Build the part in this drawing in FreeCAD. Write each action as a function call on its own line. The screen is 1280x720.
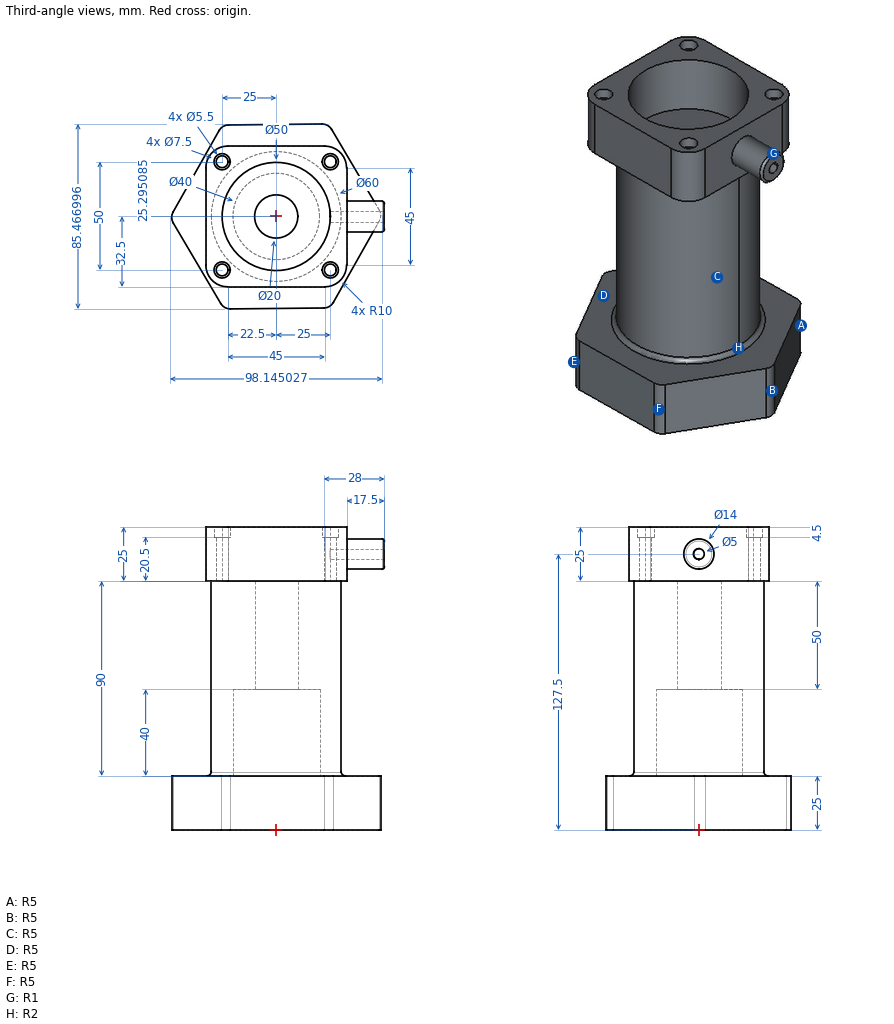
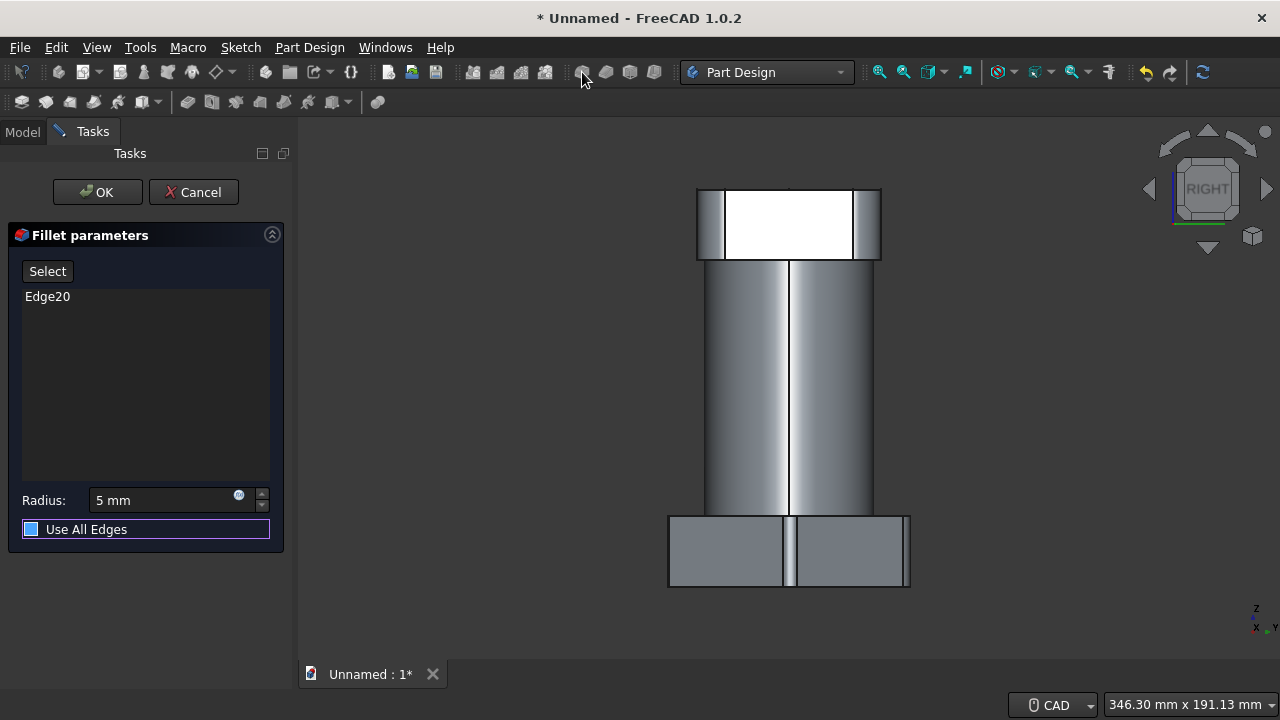
click(98, 192)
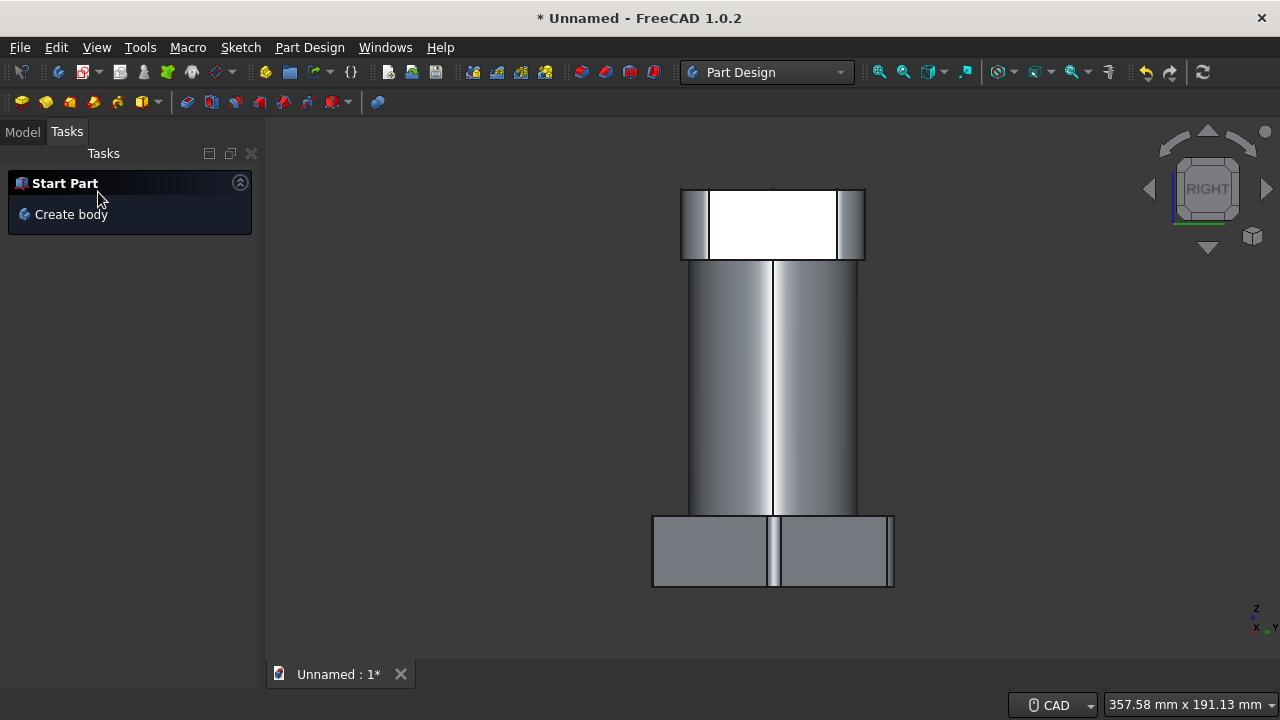
key(0)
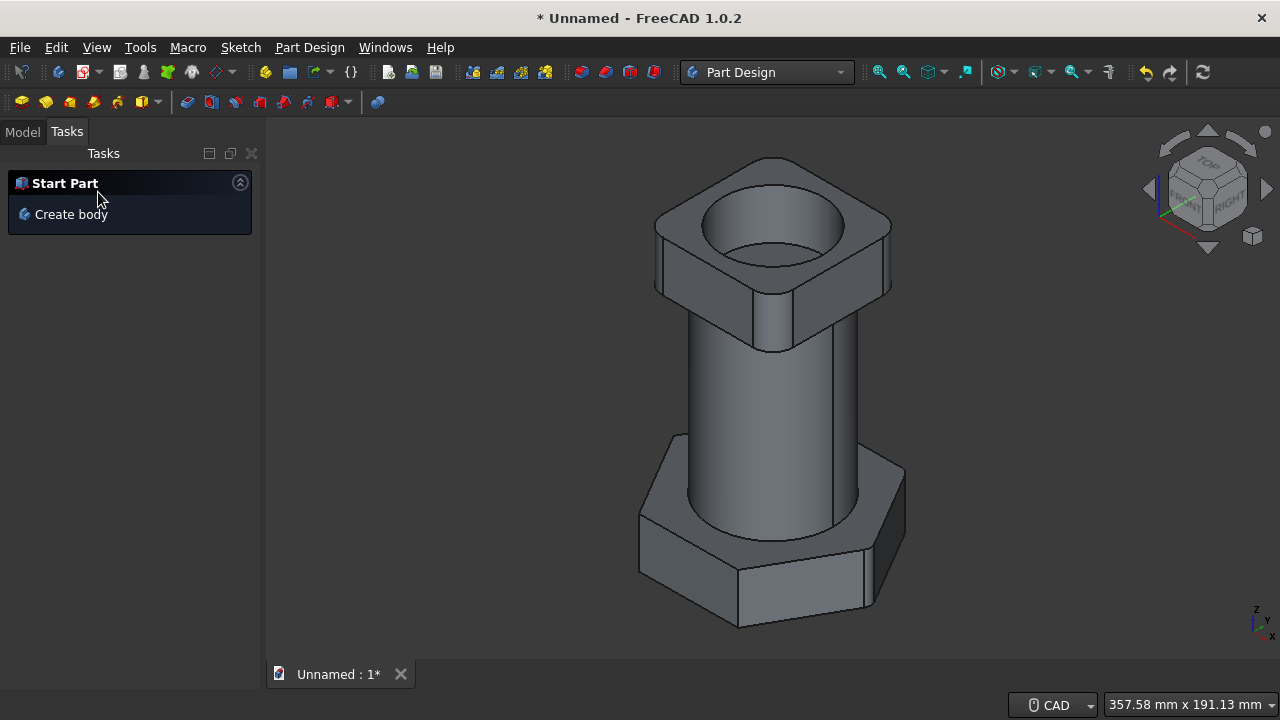
key(2)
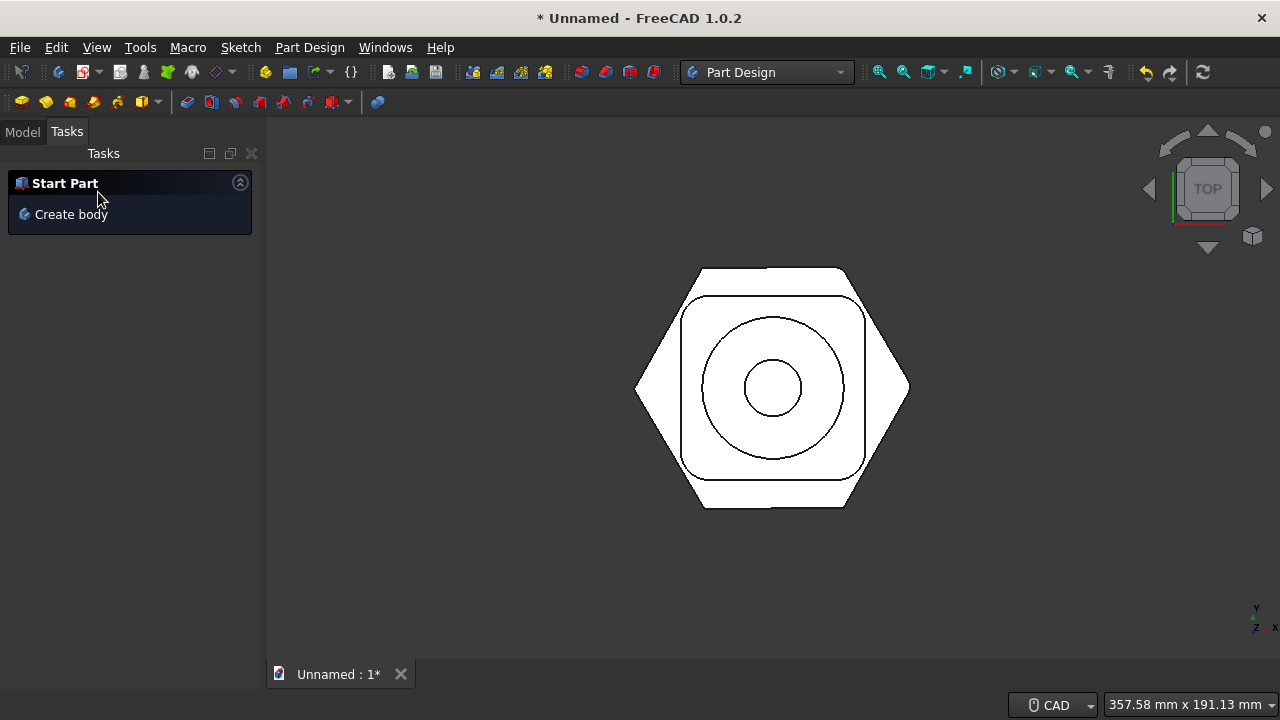
click(880, 72)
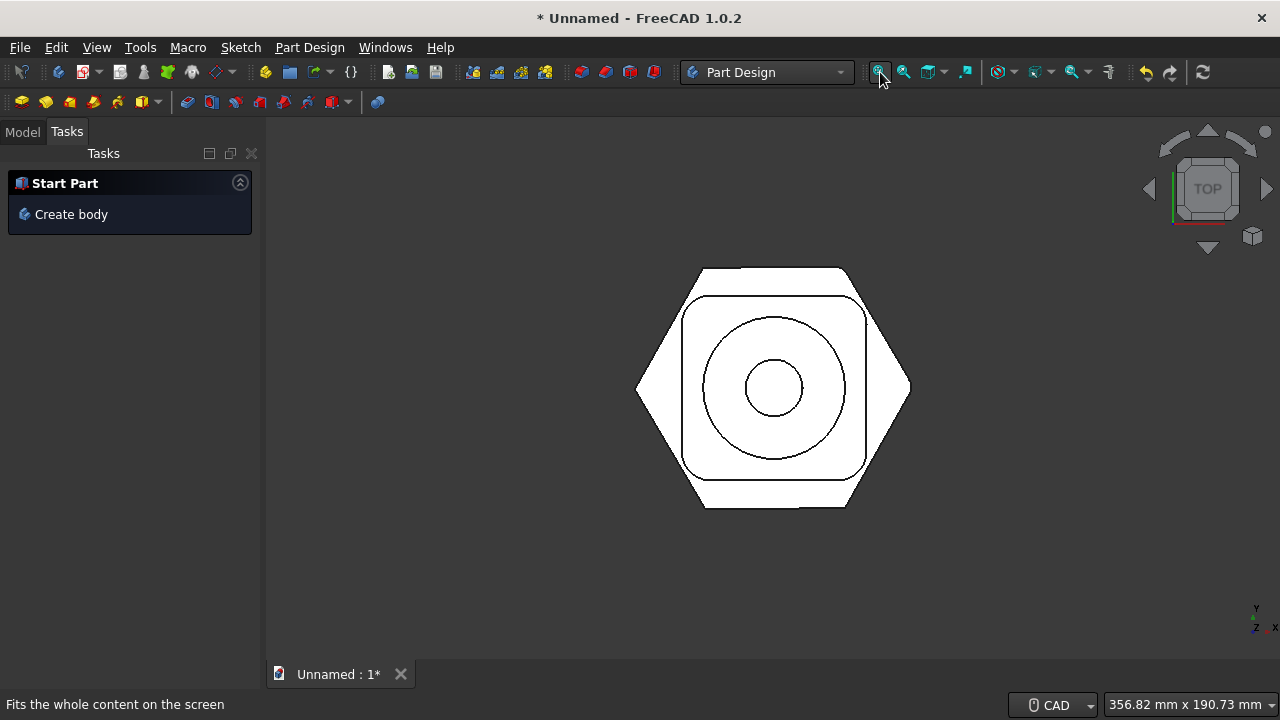
key(1)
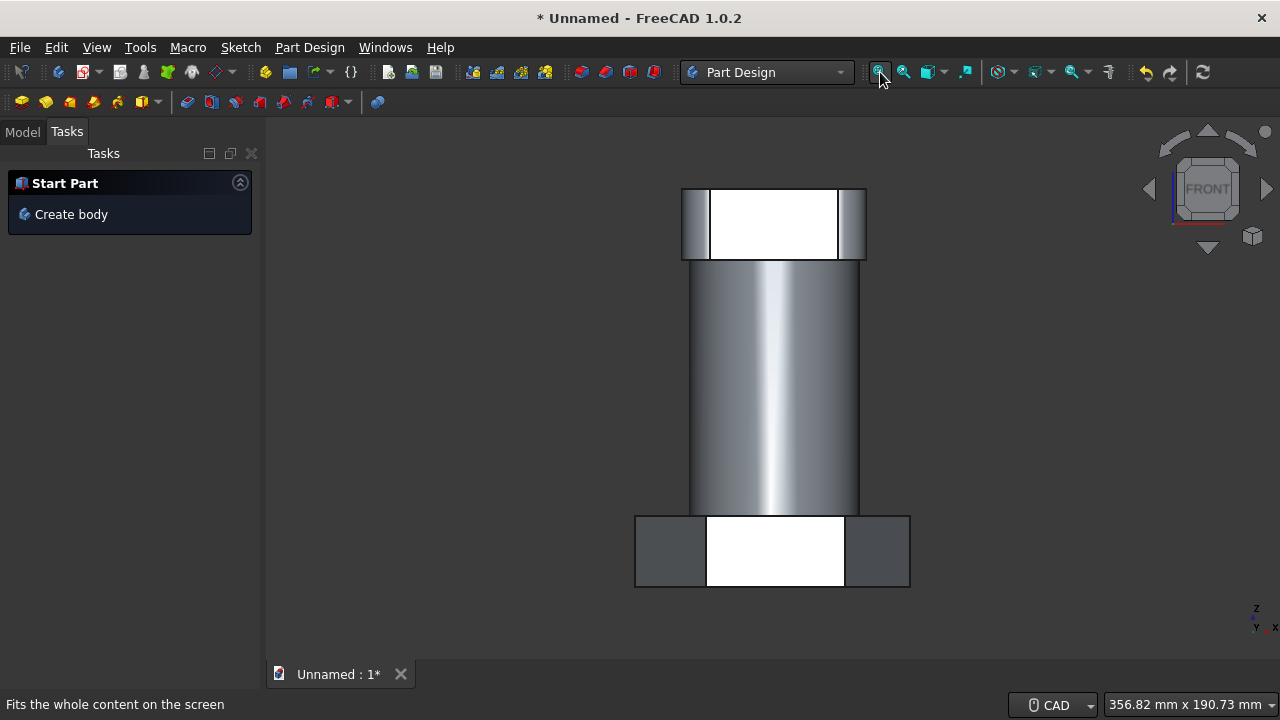
key(3)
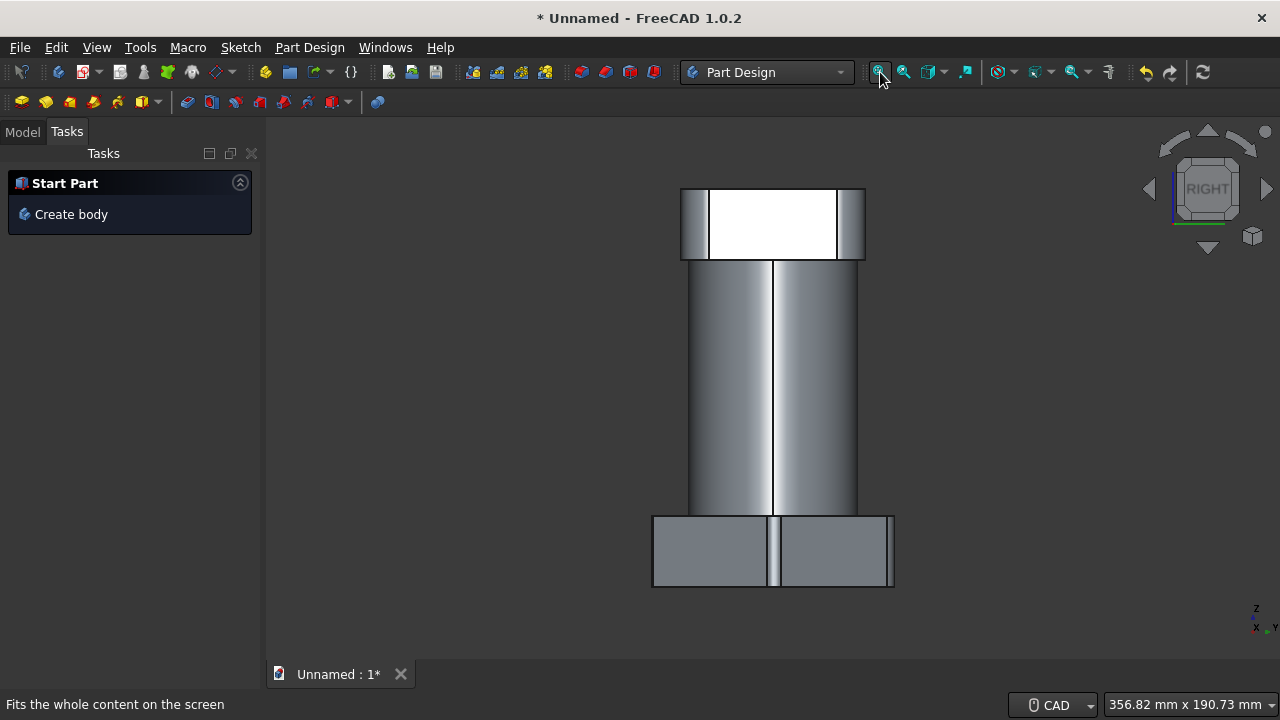
key(5)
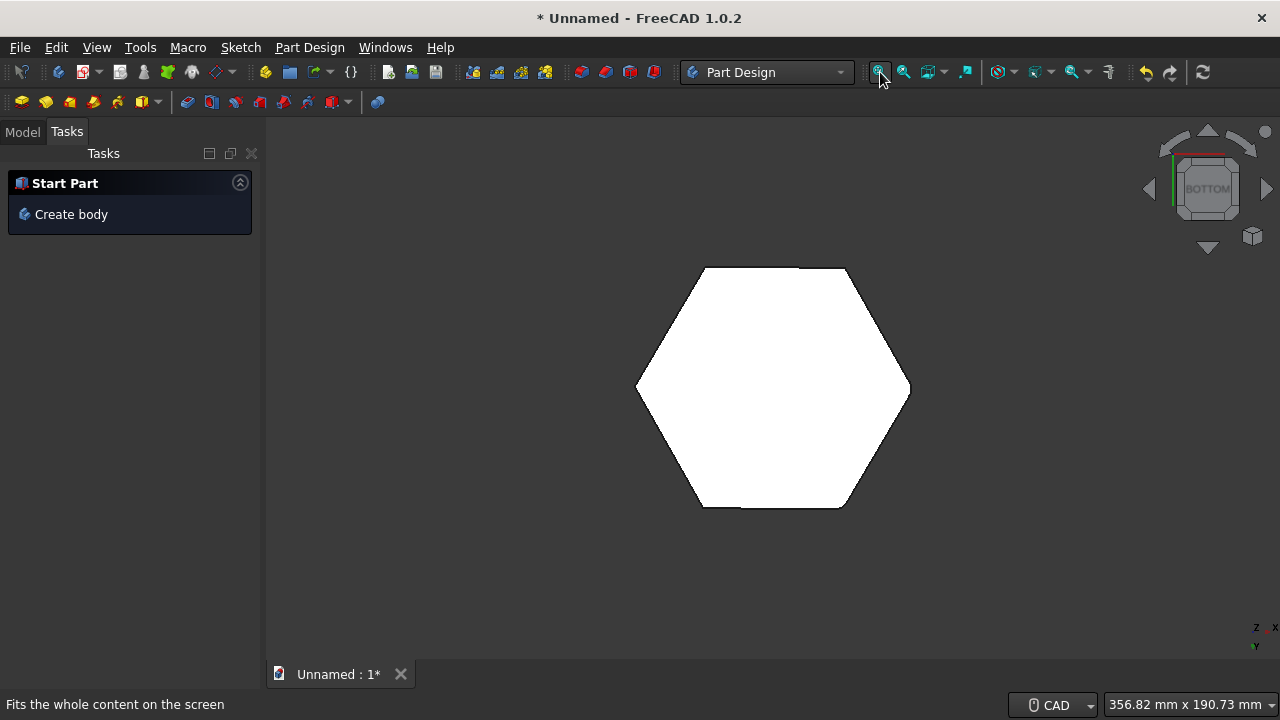
click(880, 72)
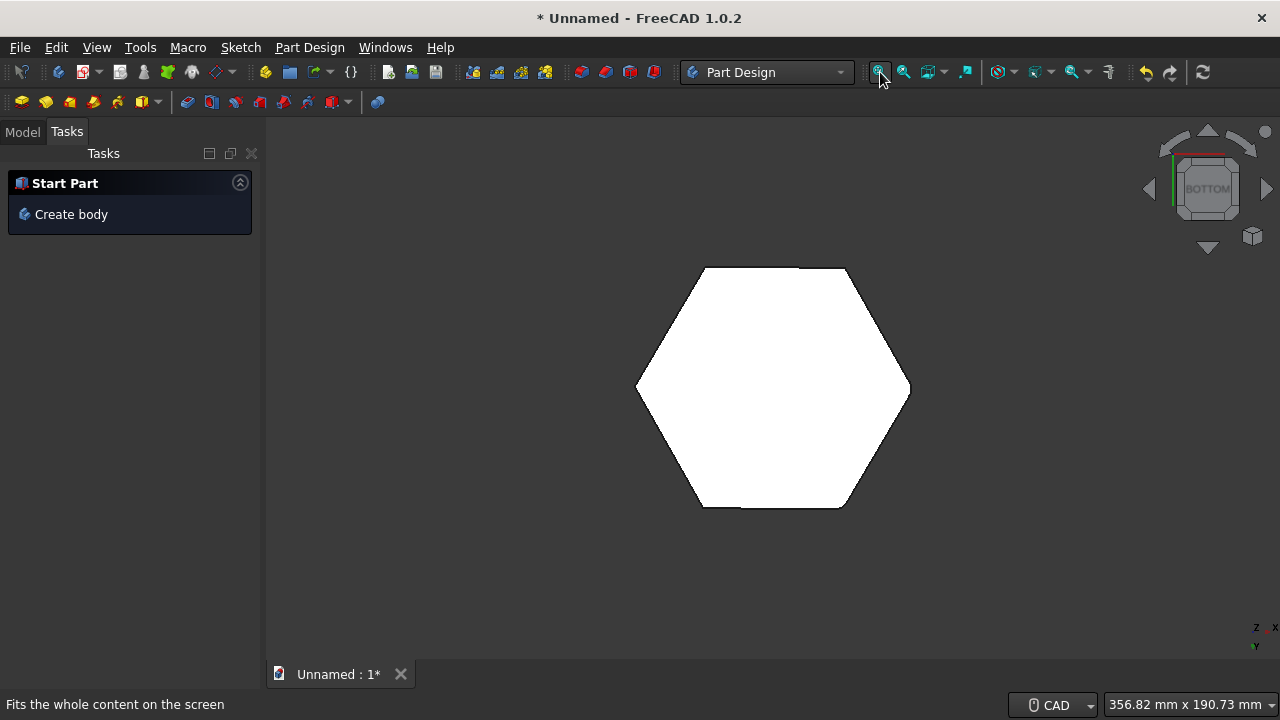
key(4)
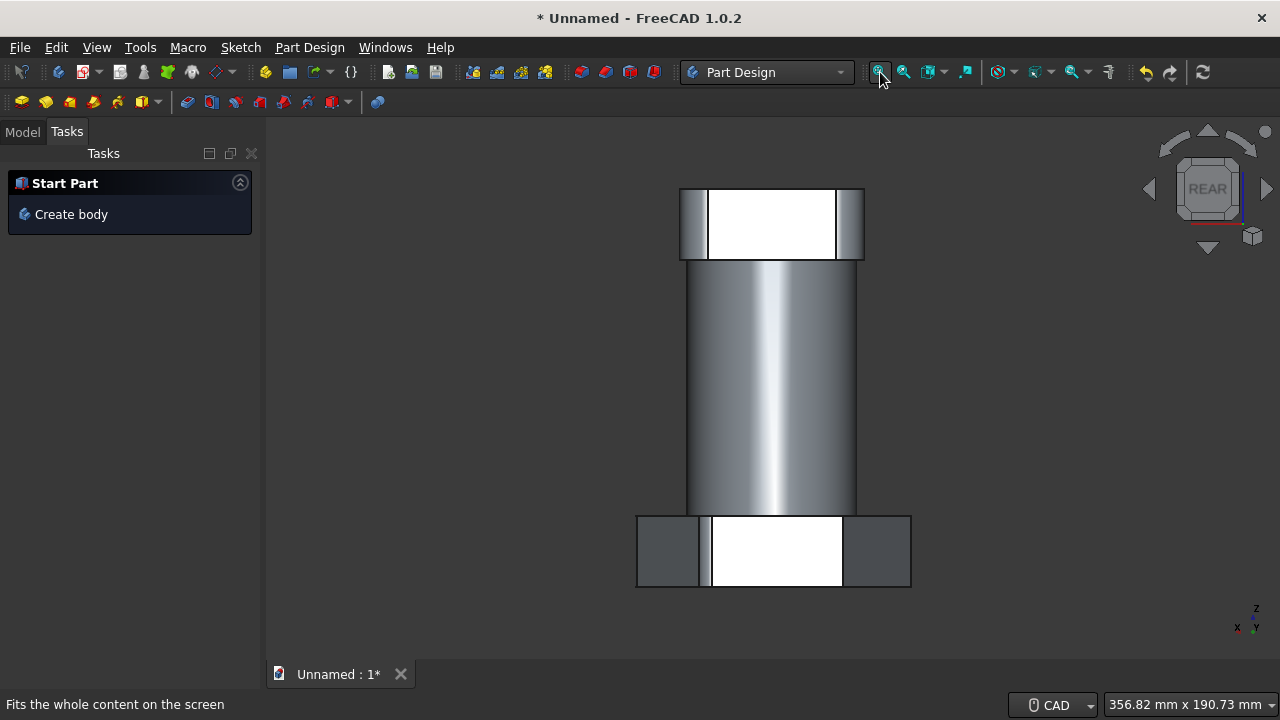
key(6)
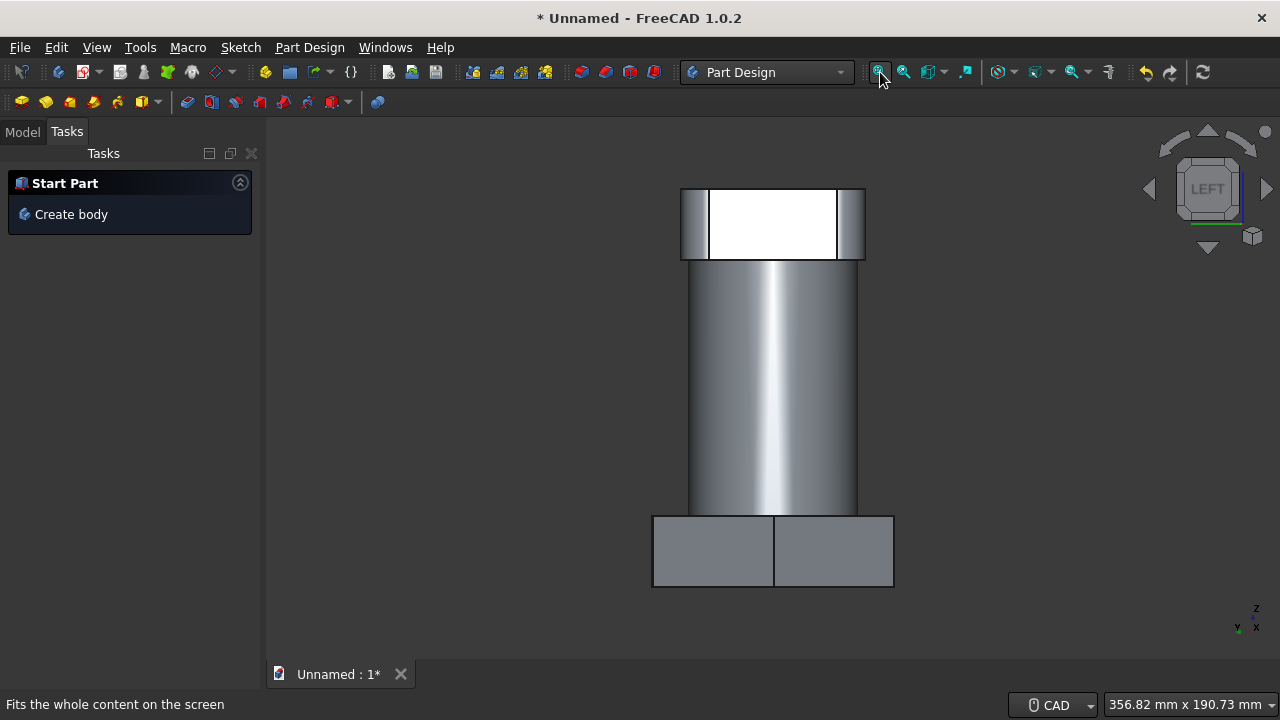
key(v)
key(3)